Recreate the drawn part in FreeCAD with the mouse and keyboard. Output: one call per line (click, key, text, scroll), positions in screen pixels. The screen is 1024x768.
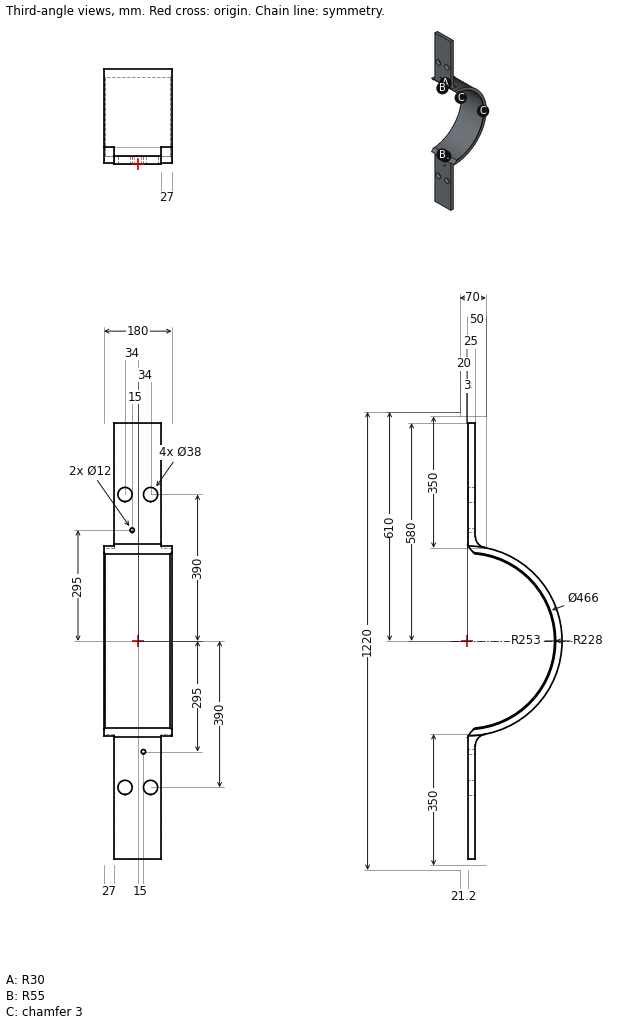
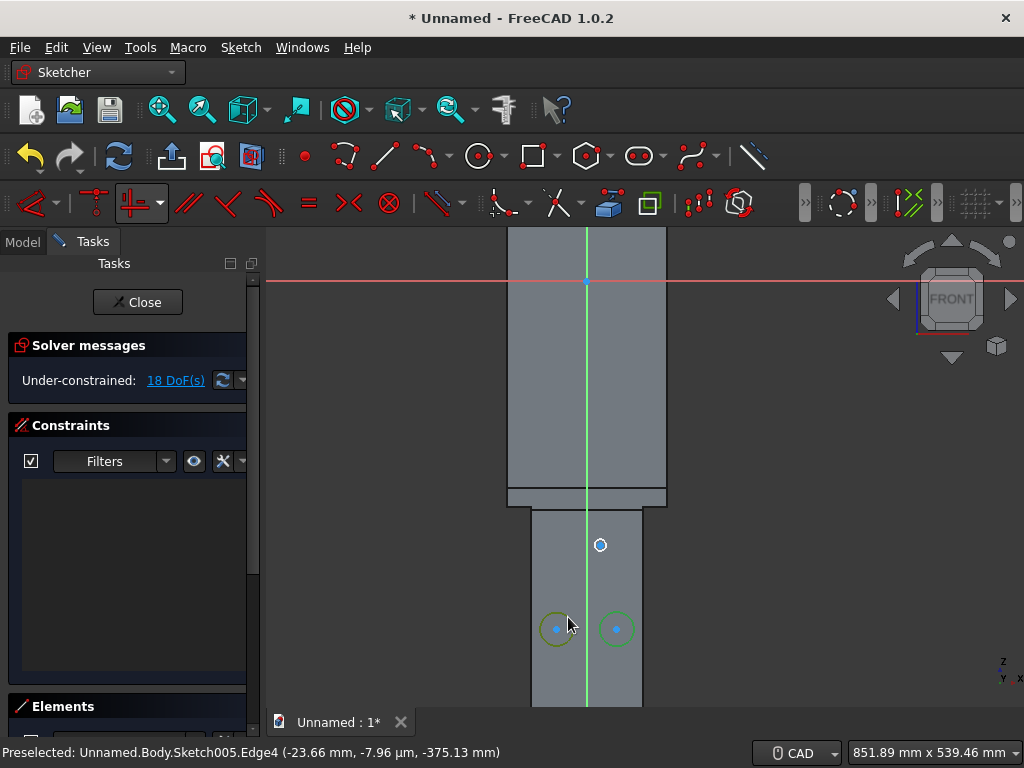
click(310, 204)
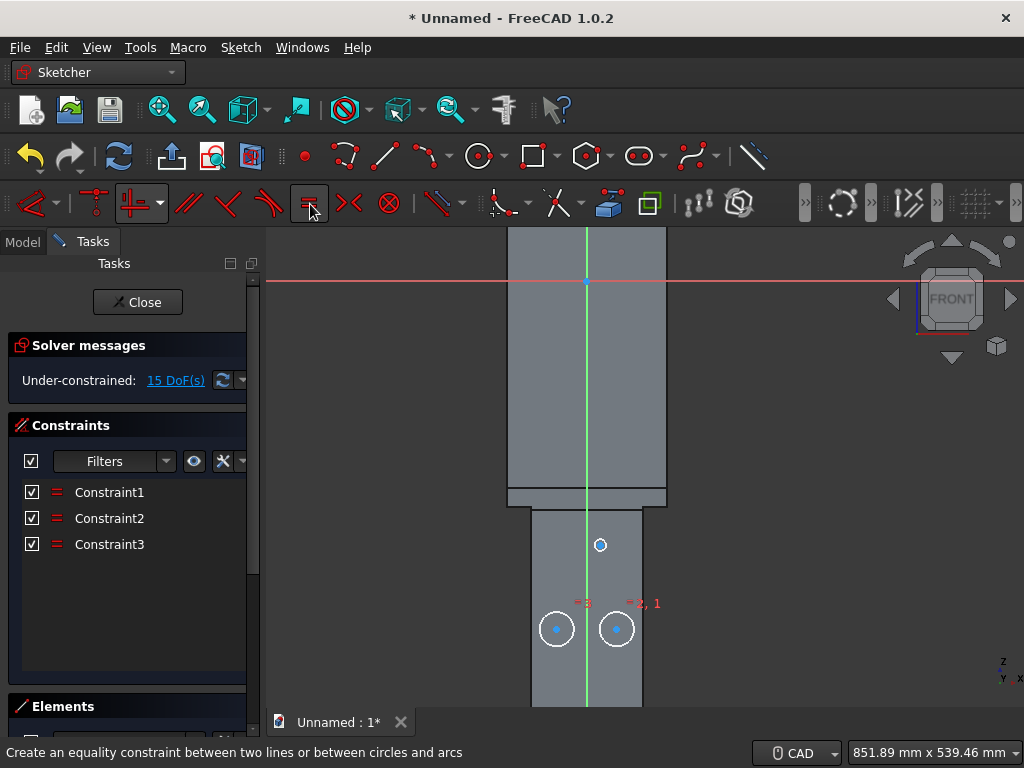
scroll(568, 618, down, 4)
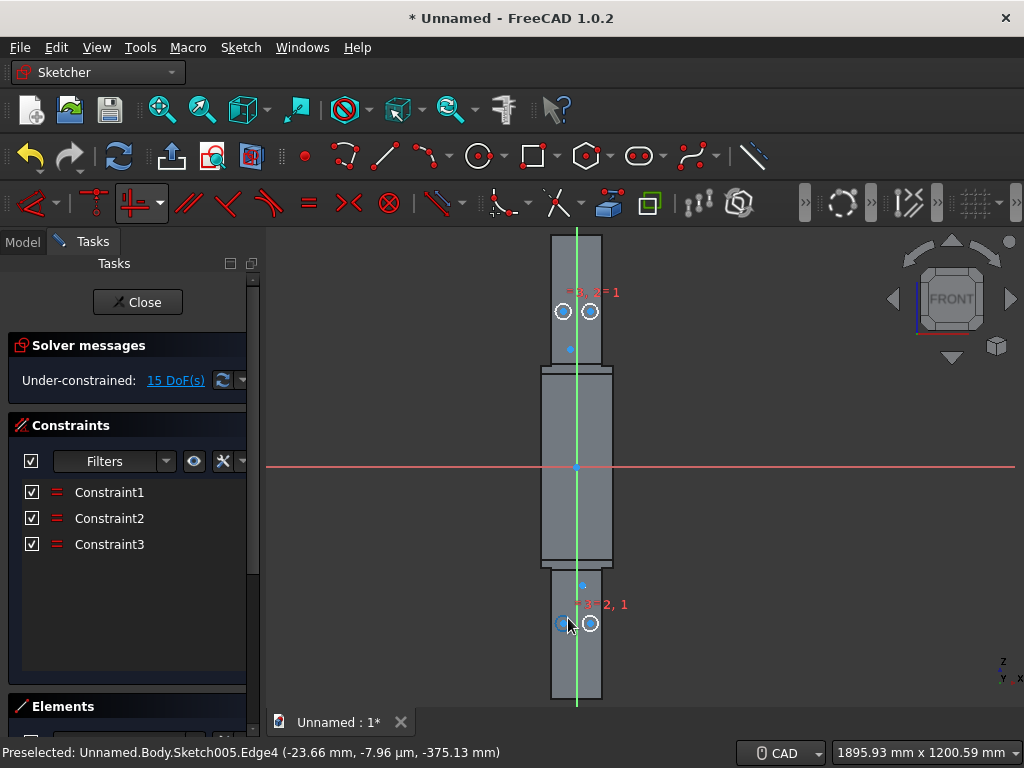
scroll(572, 348, up, 9)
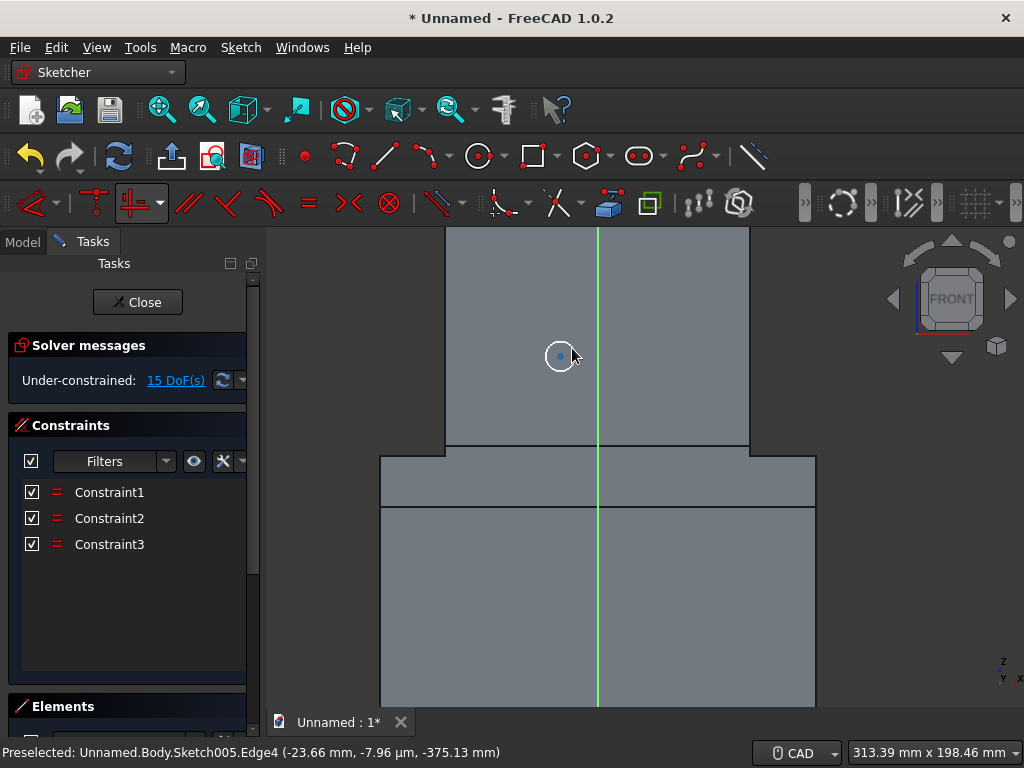
click(571, 346)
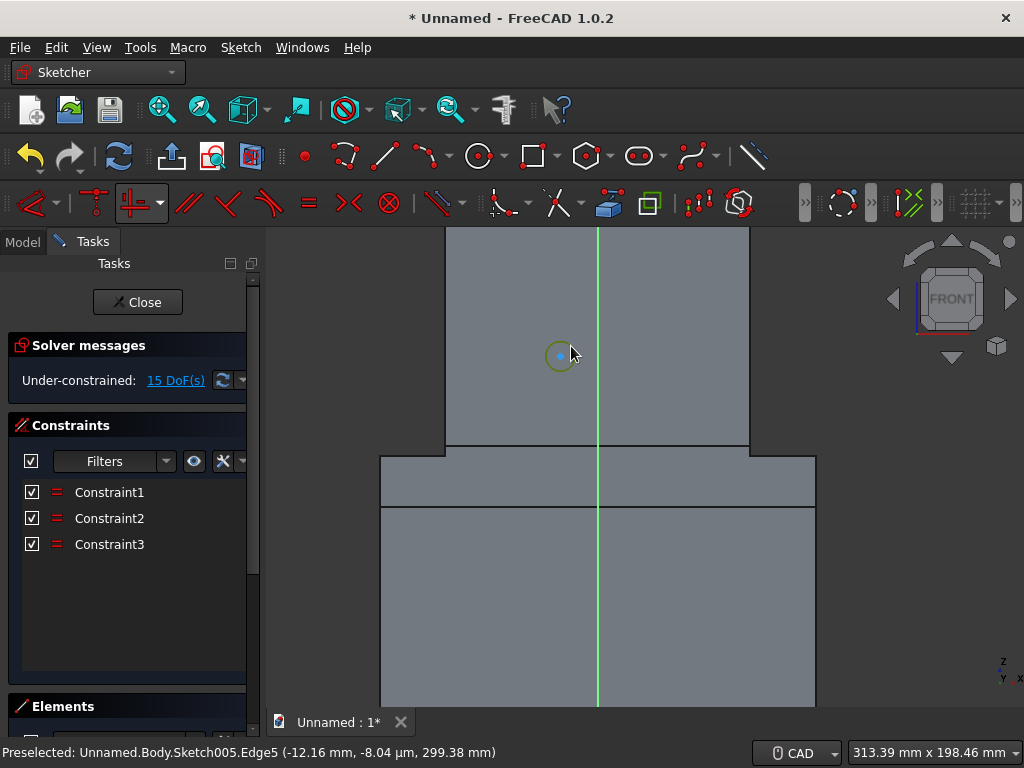
scroll(572, 348, down, 9)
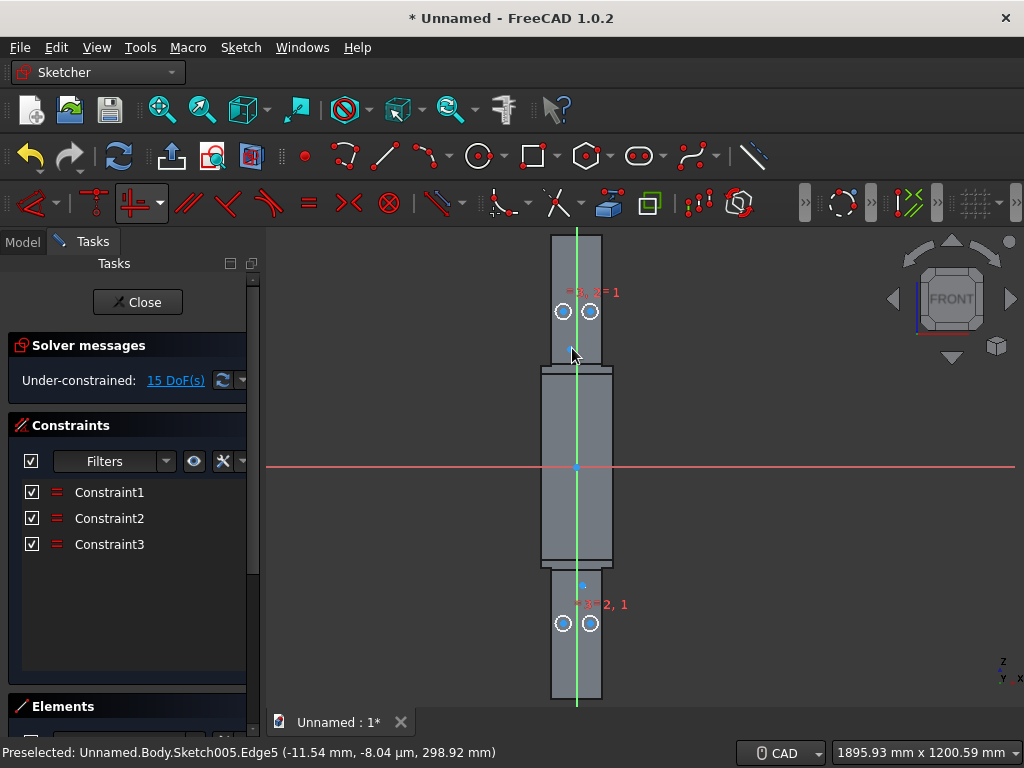
scroll(585, 584, up, 9)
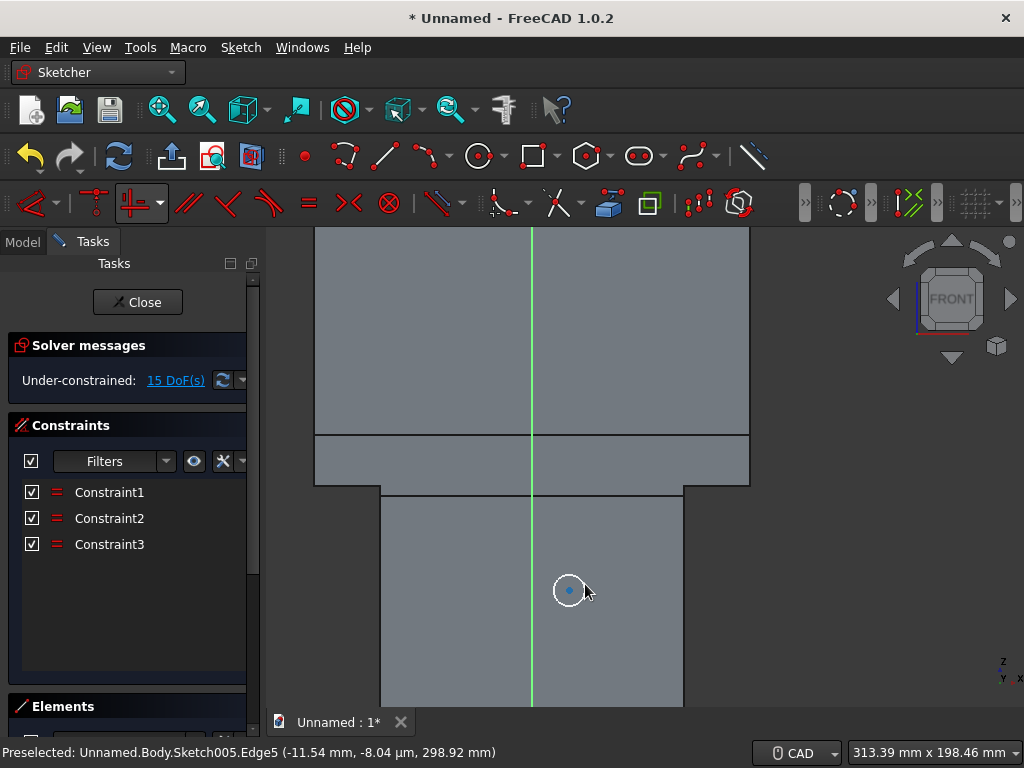
click(580, 579)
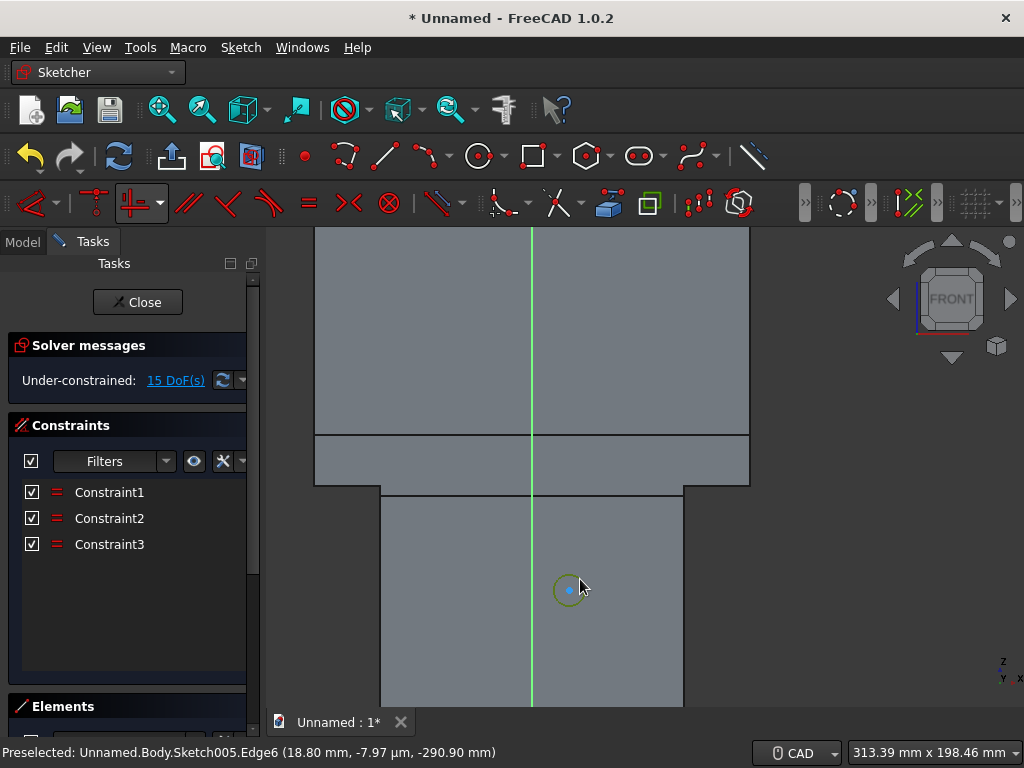
click(310, 204)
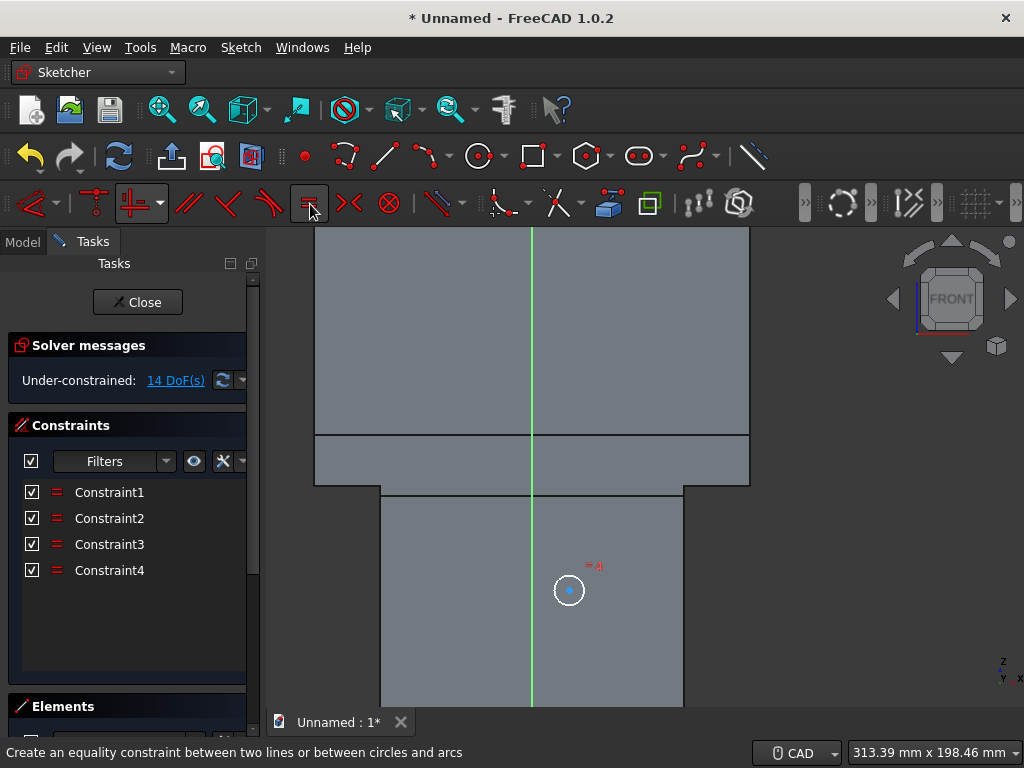
scroll(585, 584, down, 9)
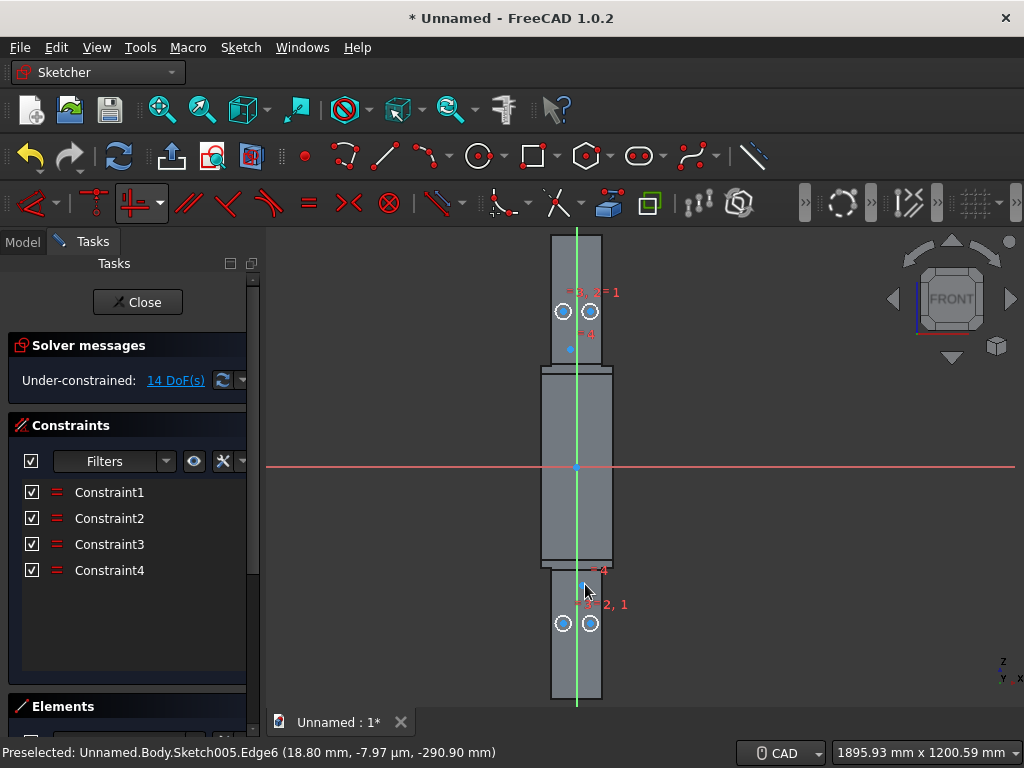
click(590, 312)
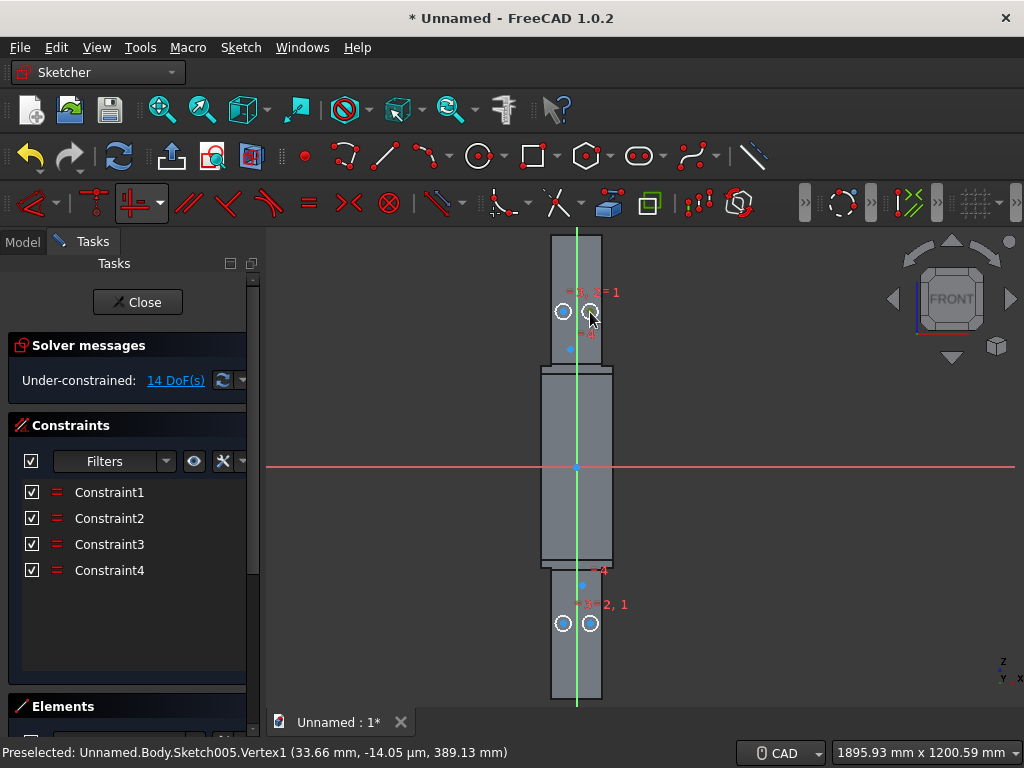
click(590, 623)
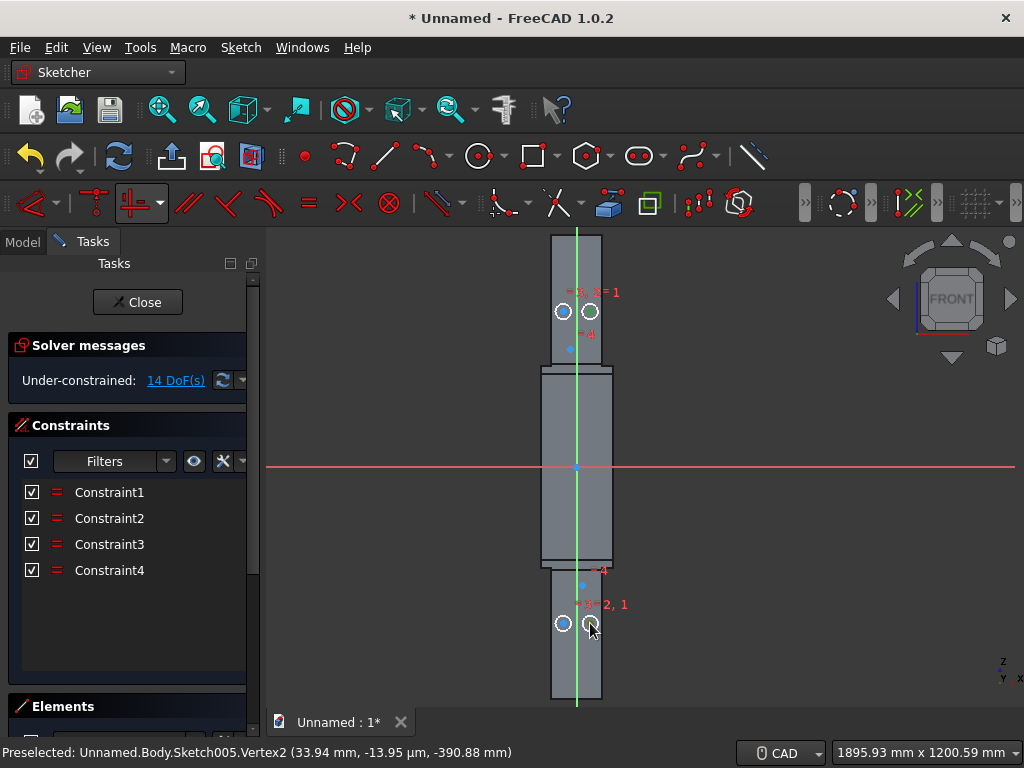
key(v)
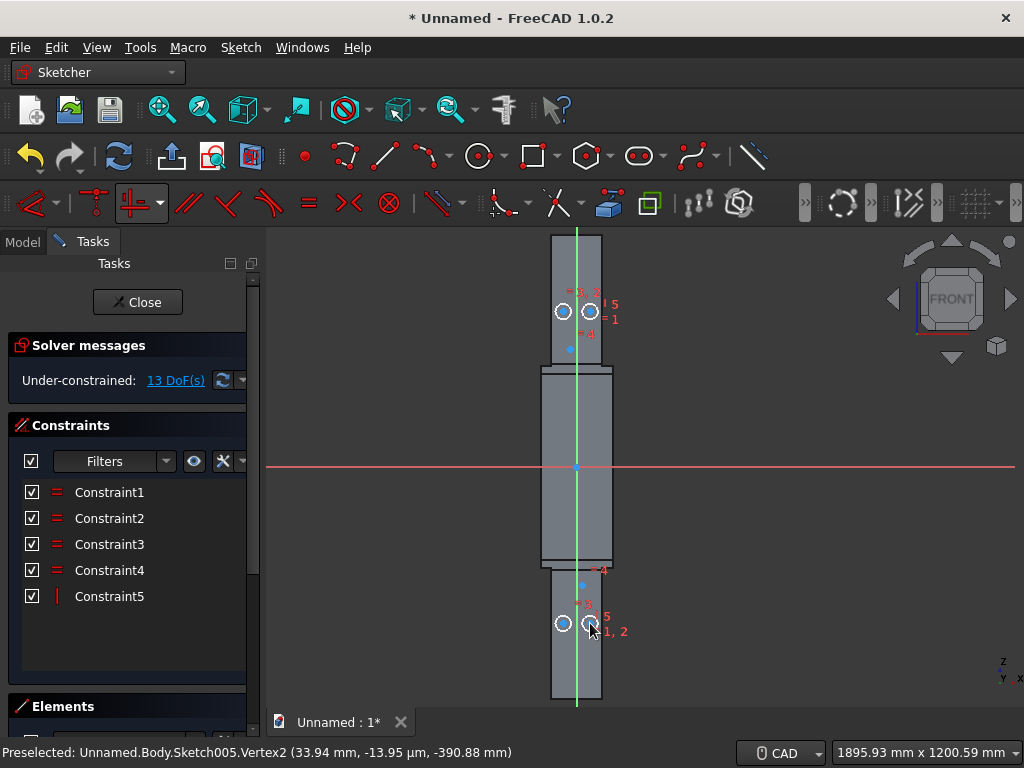
click(590, 312)